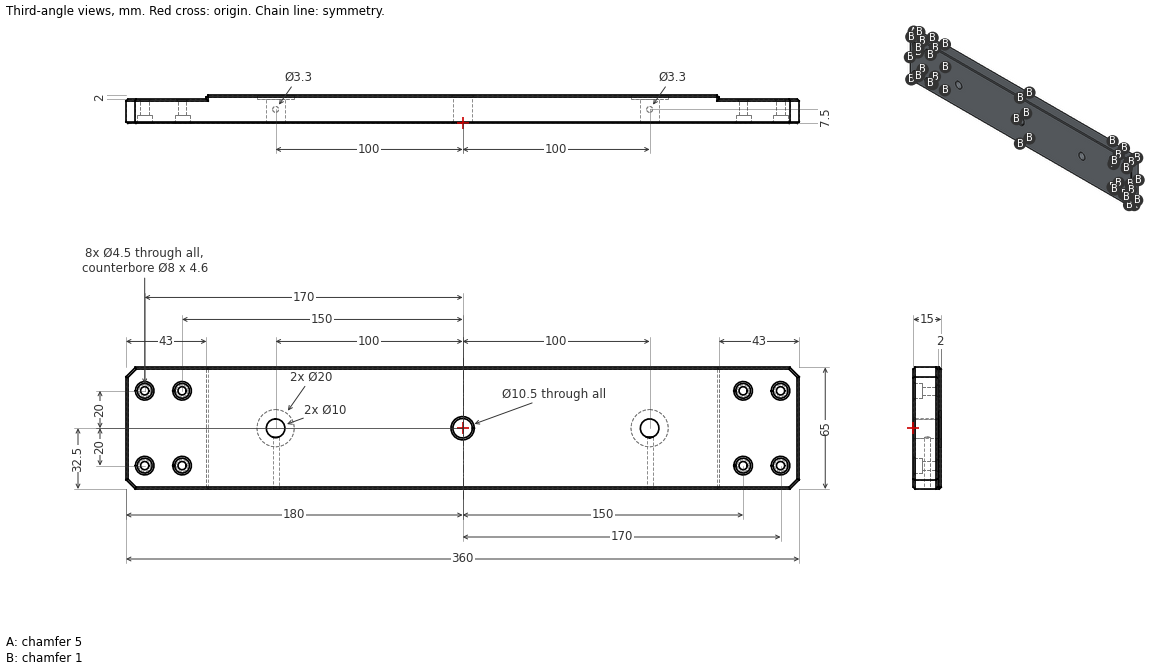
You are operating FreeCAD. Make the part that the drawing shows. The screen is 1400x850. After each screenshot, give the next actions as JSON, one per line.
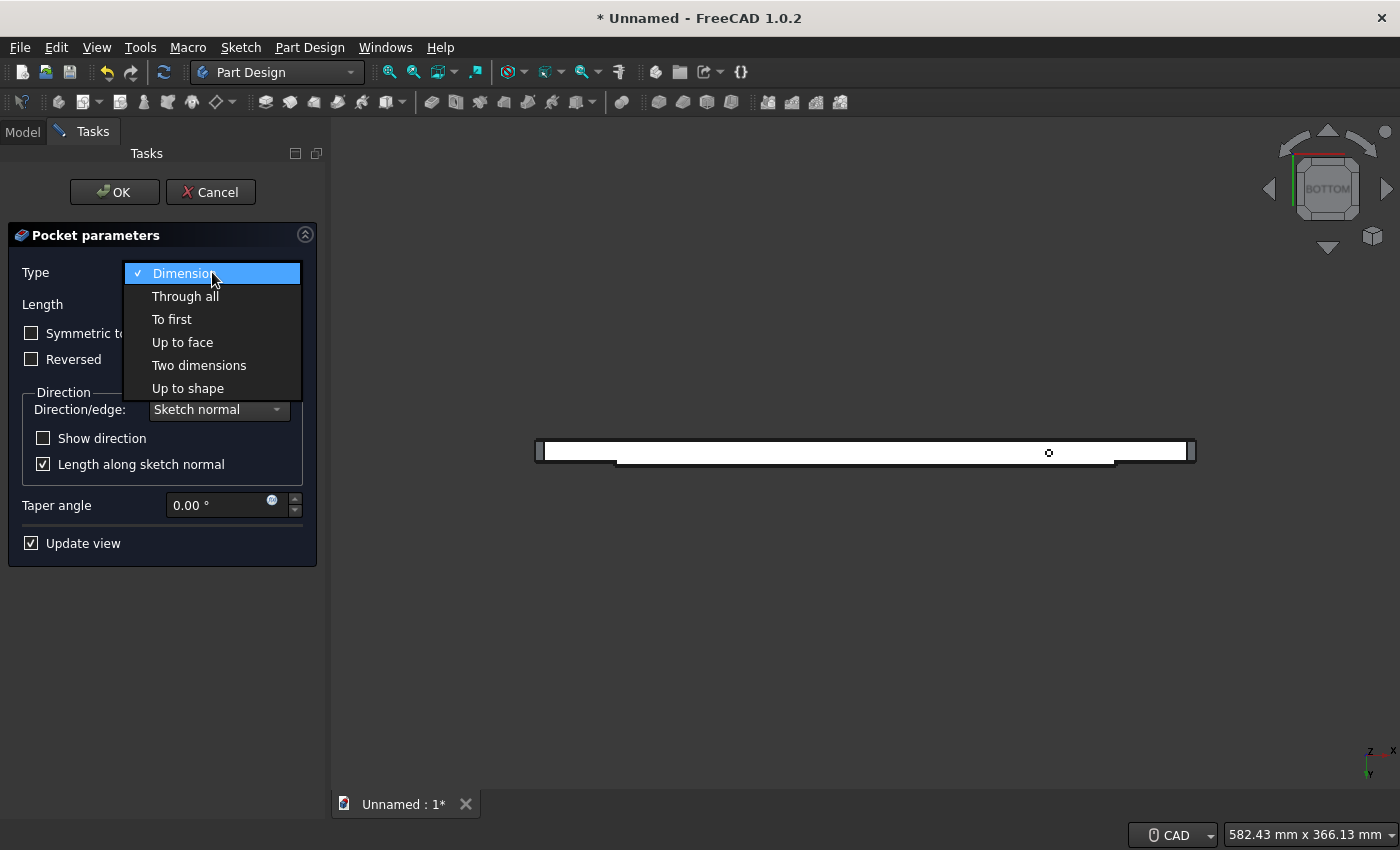
{"action": "left_click", "coordinate": [212, 320]}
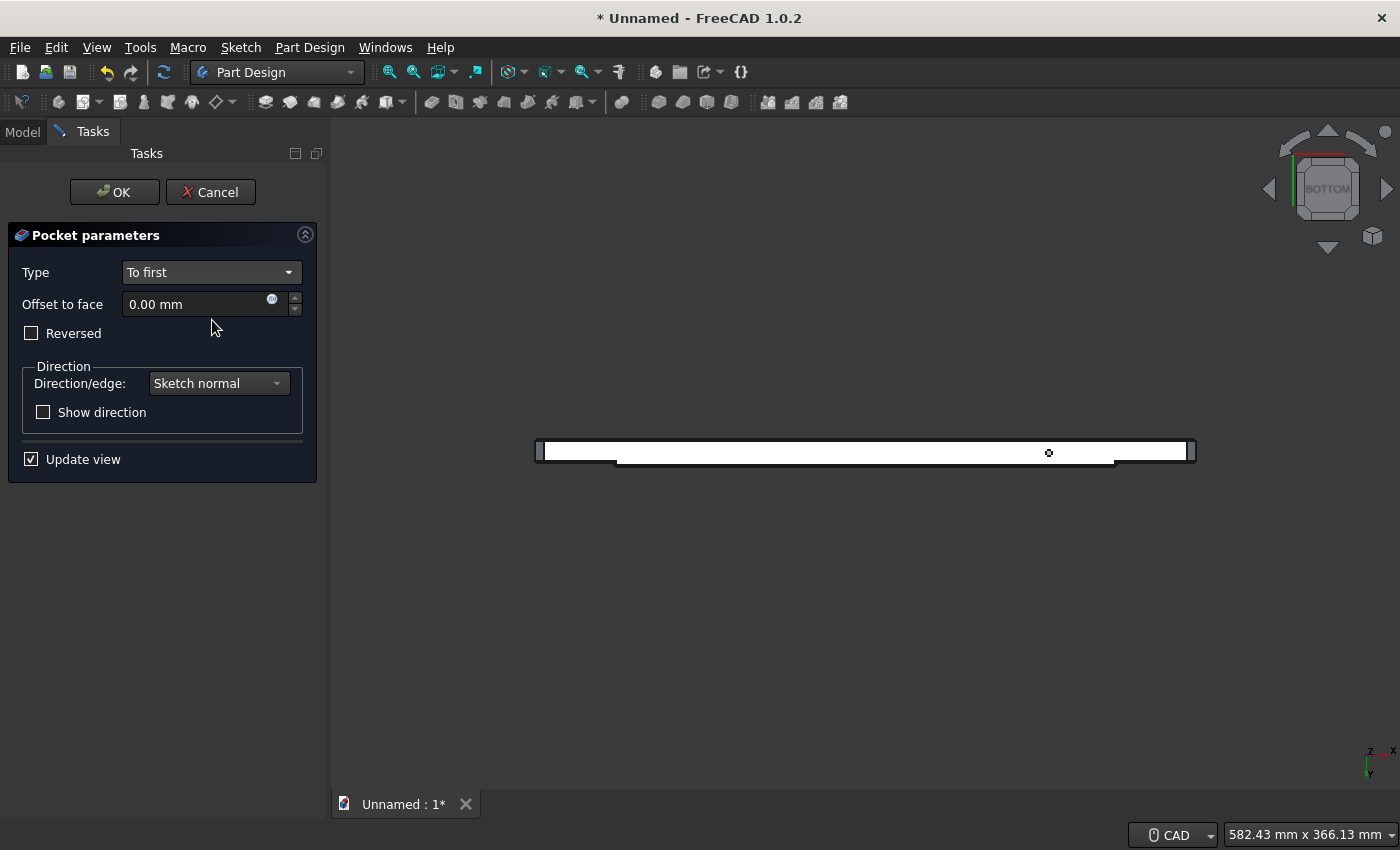
{"action": "left_click", "coordinate": [115, 192]}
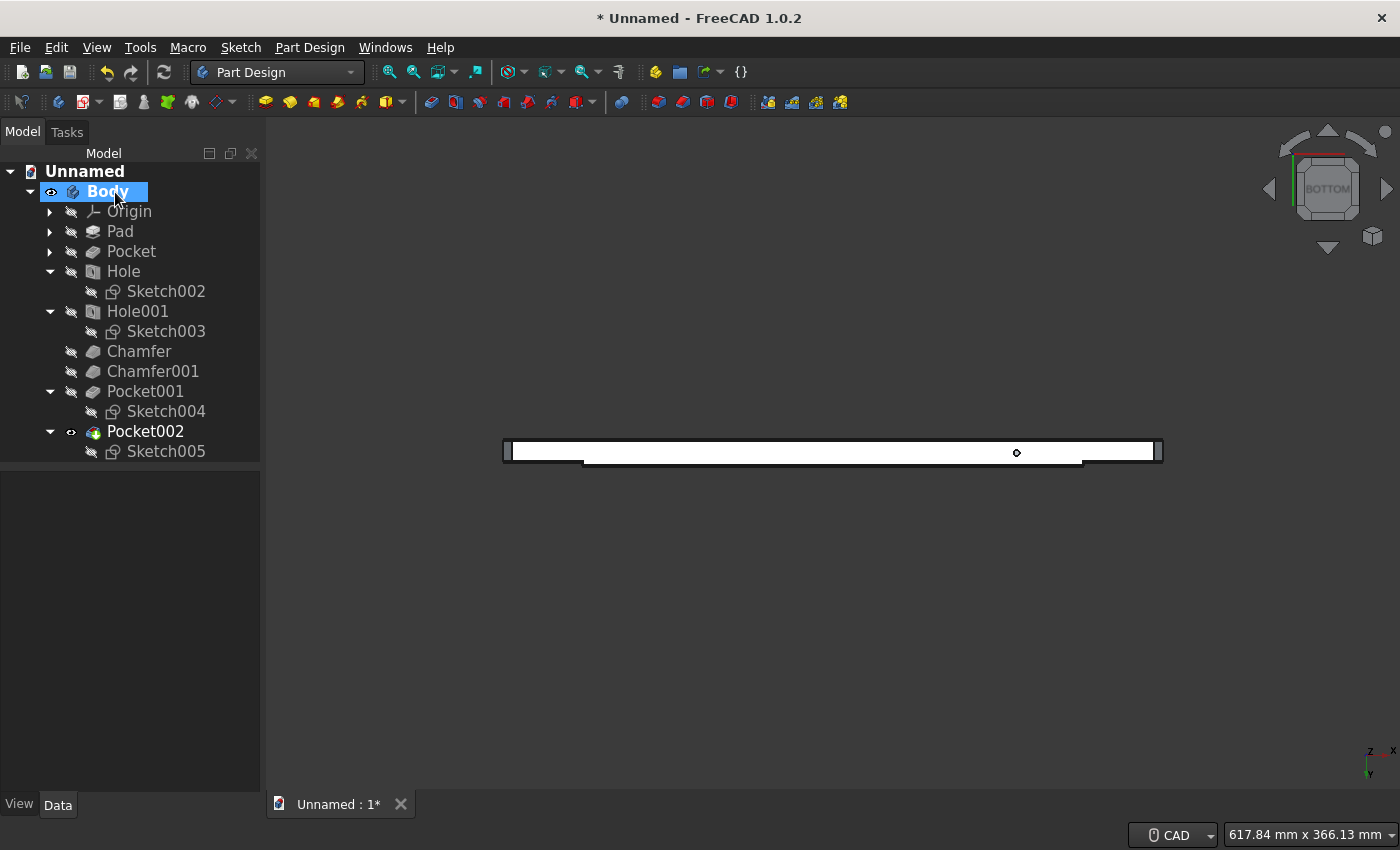
{"action": "left_click", "coordinate": [925, 452]}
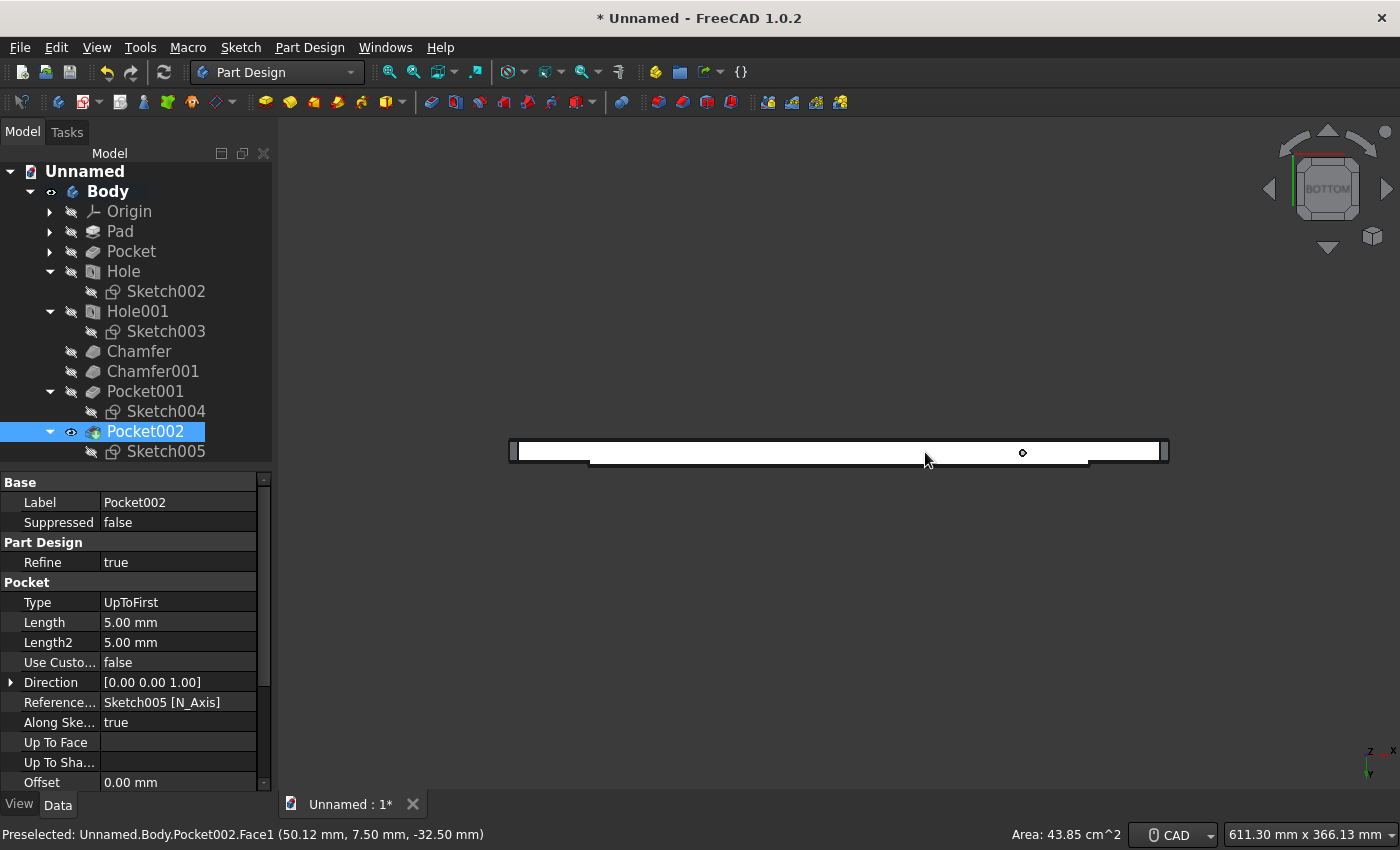
{"action": "left_click", "coordinate": [84, 102]}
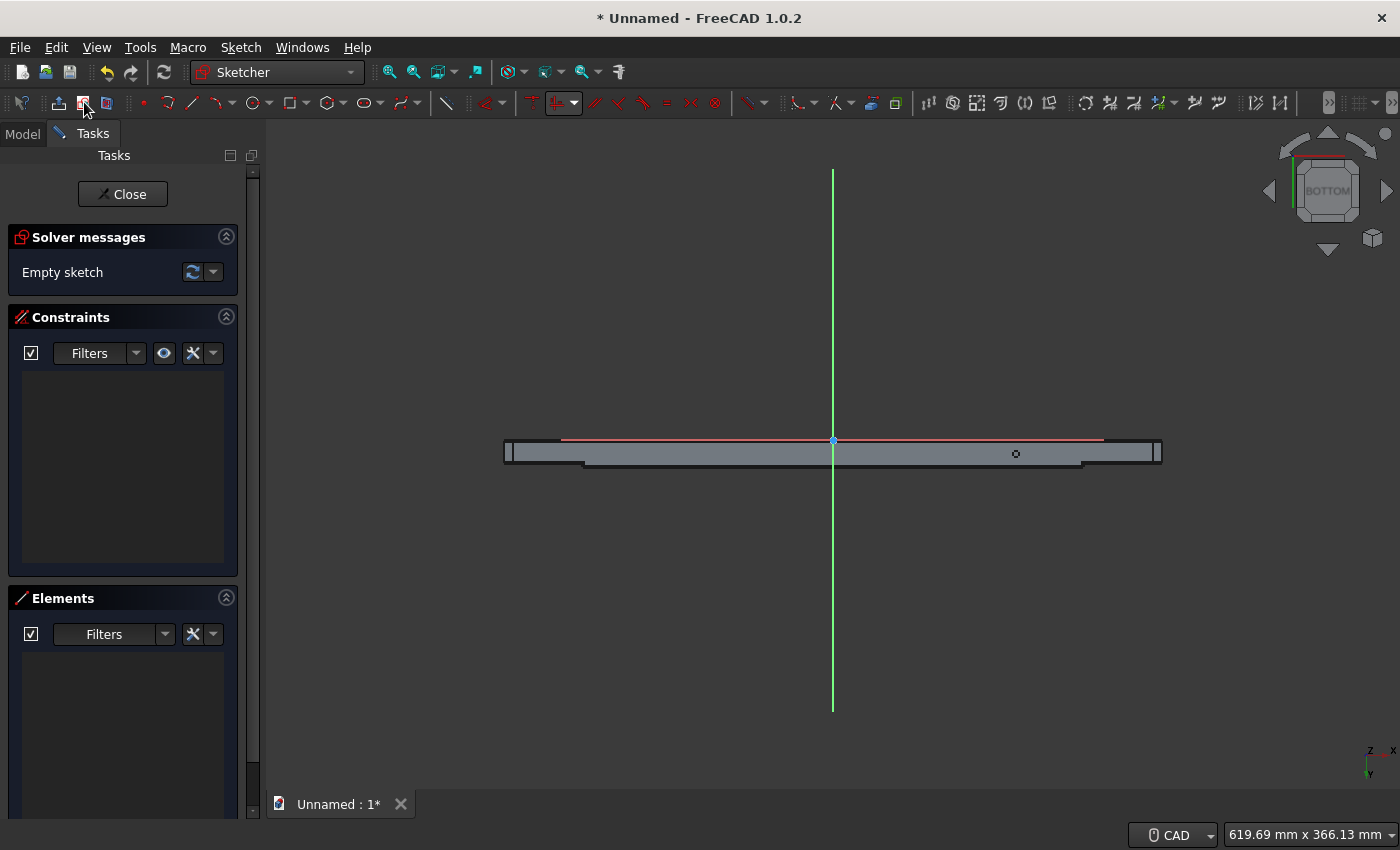
{"action": "scroll", "coordinate": [644, 454], "scroll_direction": "up", "scroll_amount": 15}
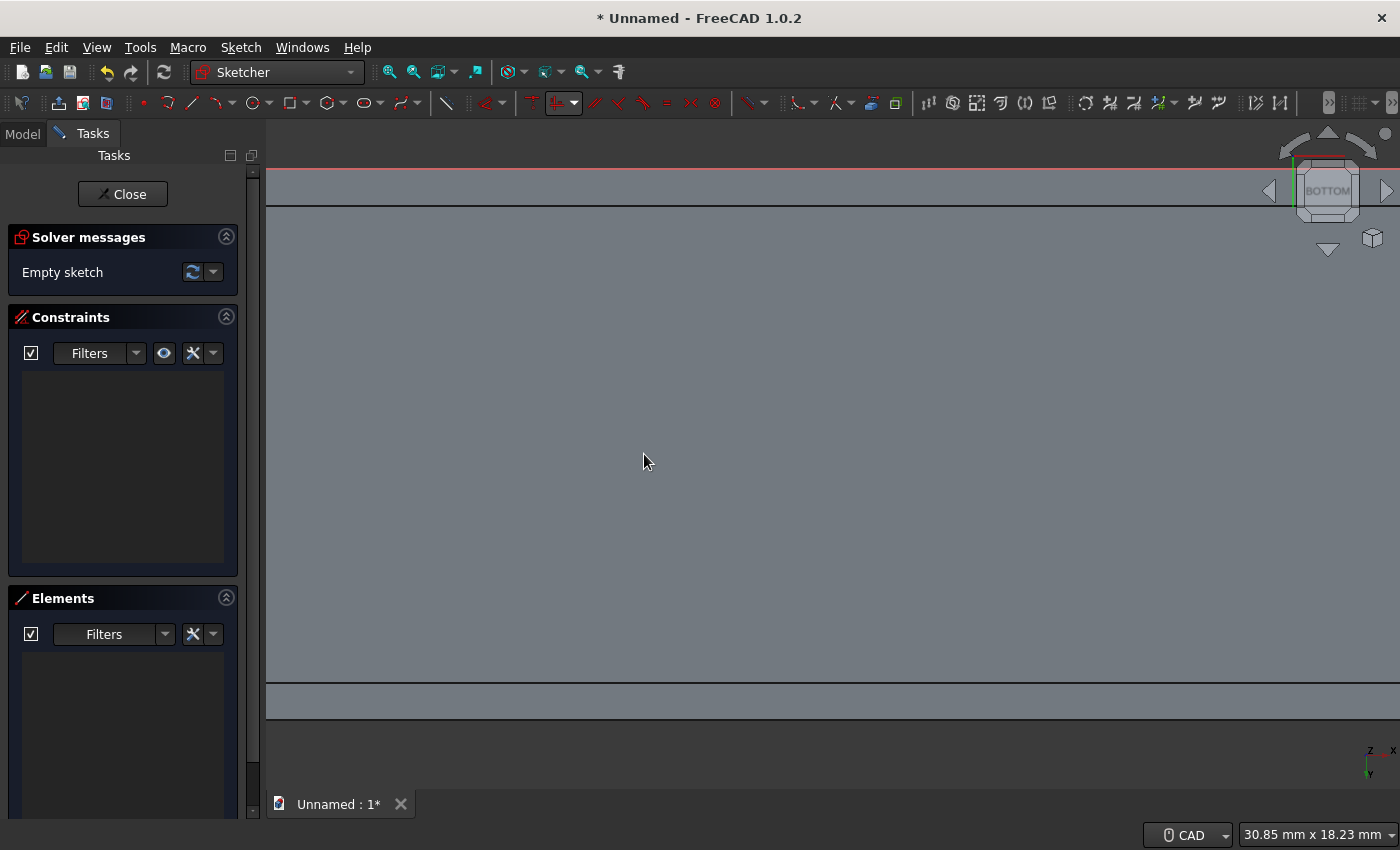
{"action": "scroll", "coordinate": [756, 440], "scroll_direction": "up", "scroll_amount": 6}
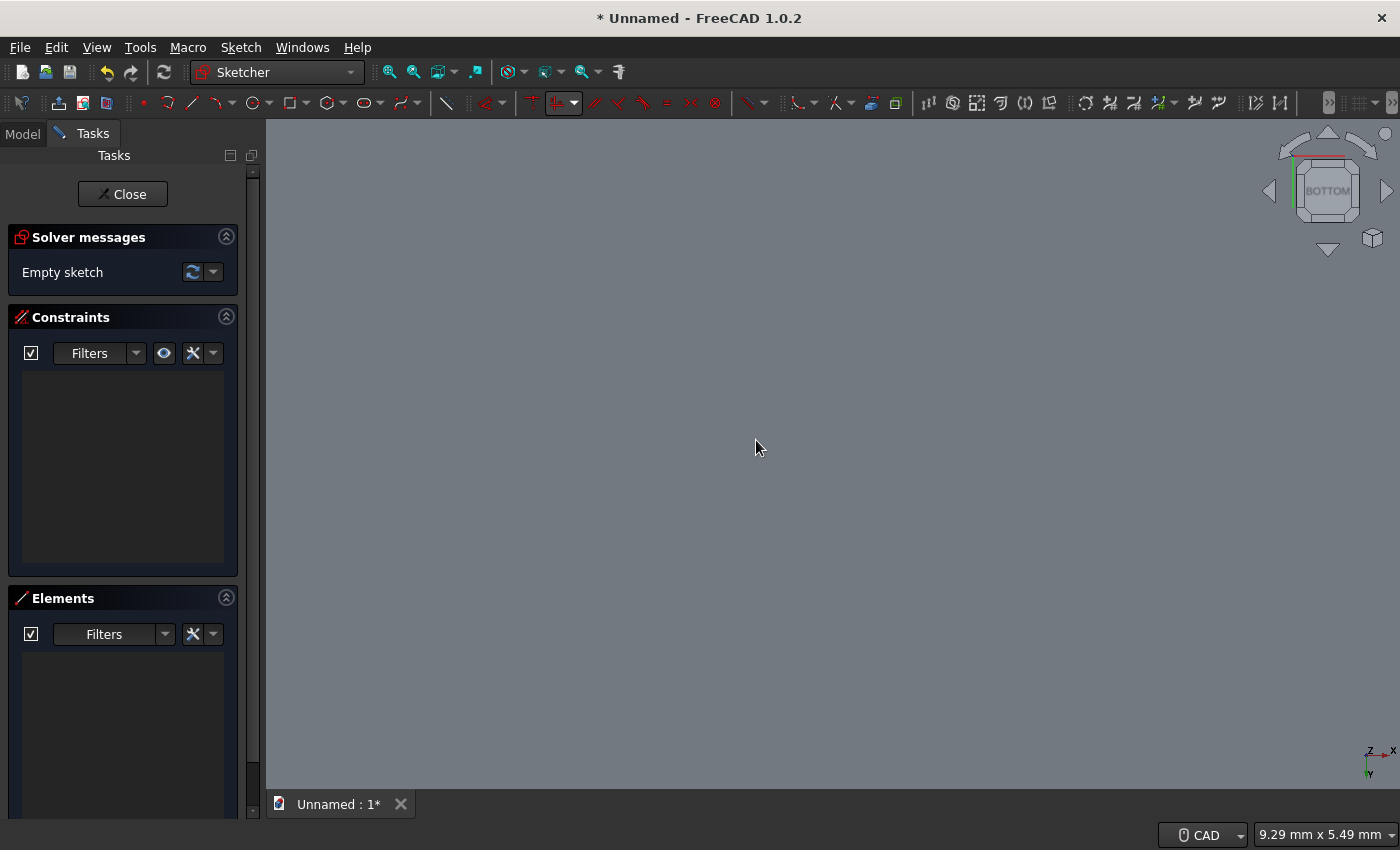
{"action": "left_click", "coordinate": [254, 104]}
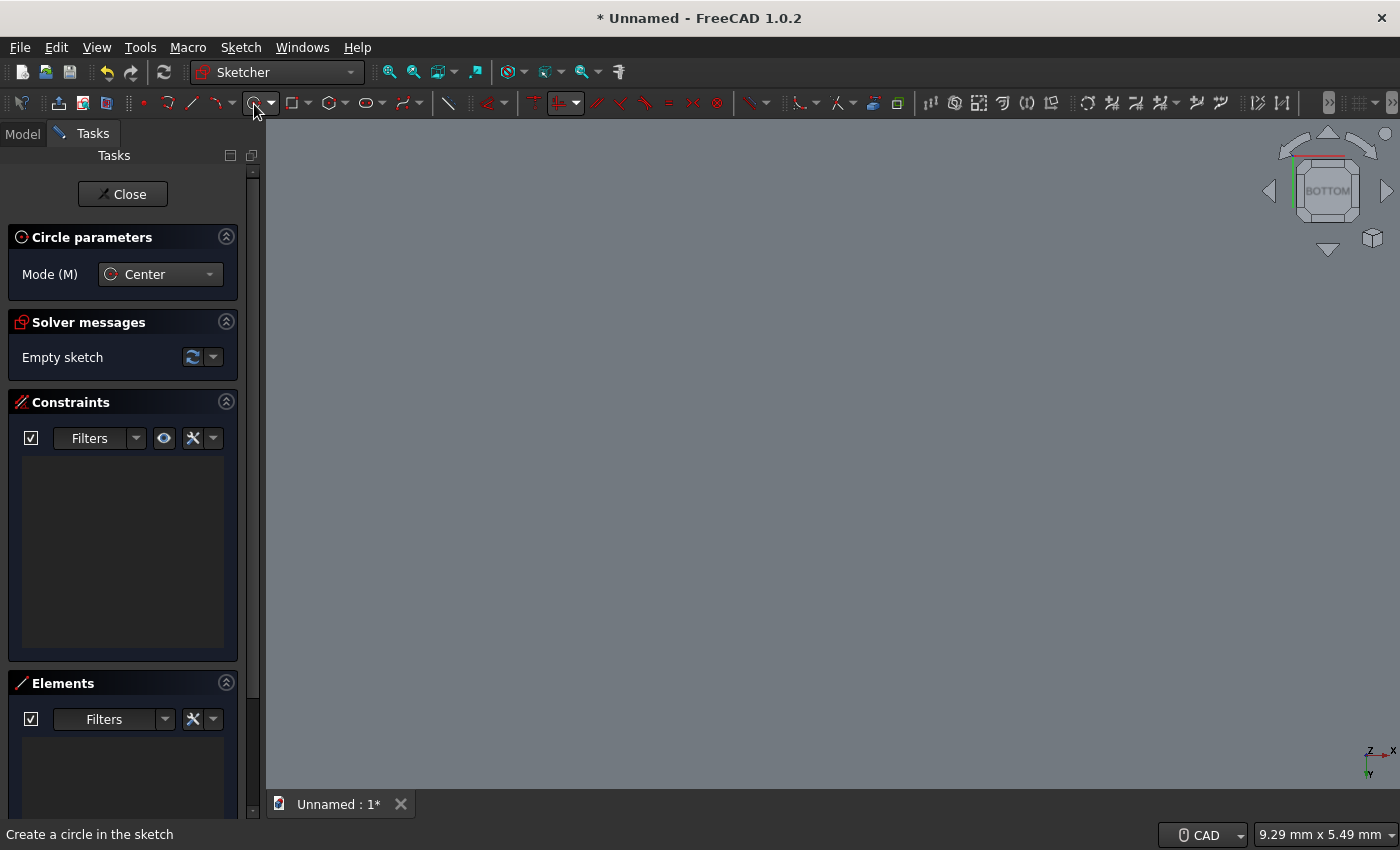
{"action": "left_click", "coordinate": [762, 454]}
{"action": "mouse_move", "coordinate": [905, 311]}